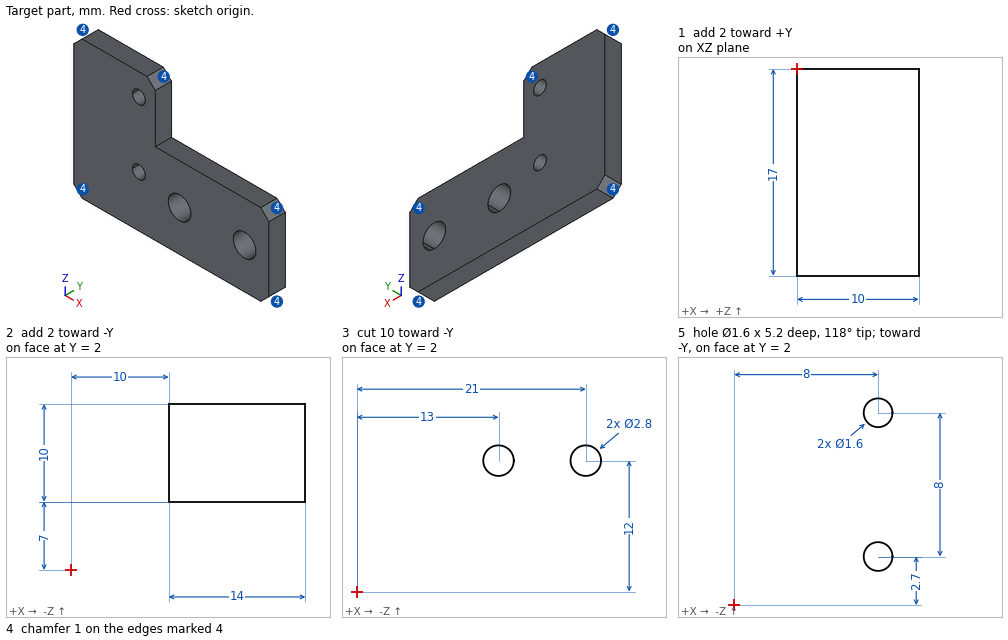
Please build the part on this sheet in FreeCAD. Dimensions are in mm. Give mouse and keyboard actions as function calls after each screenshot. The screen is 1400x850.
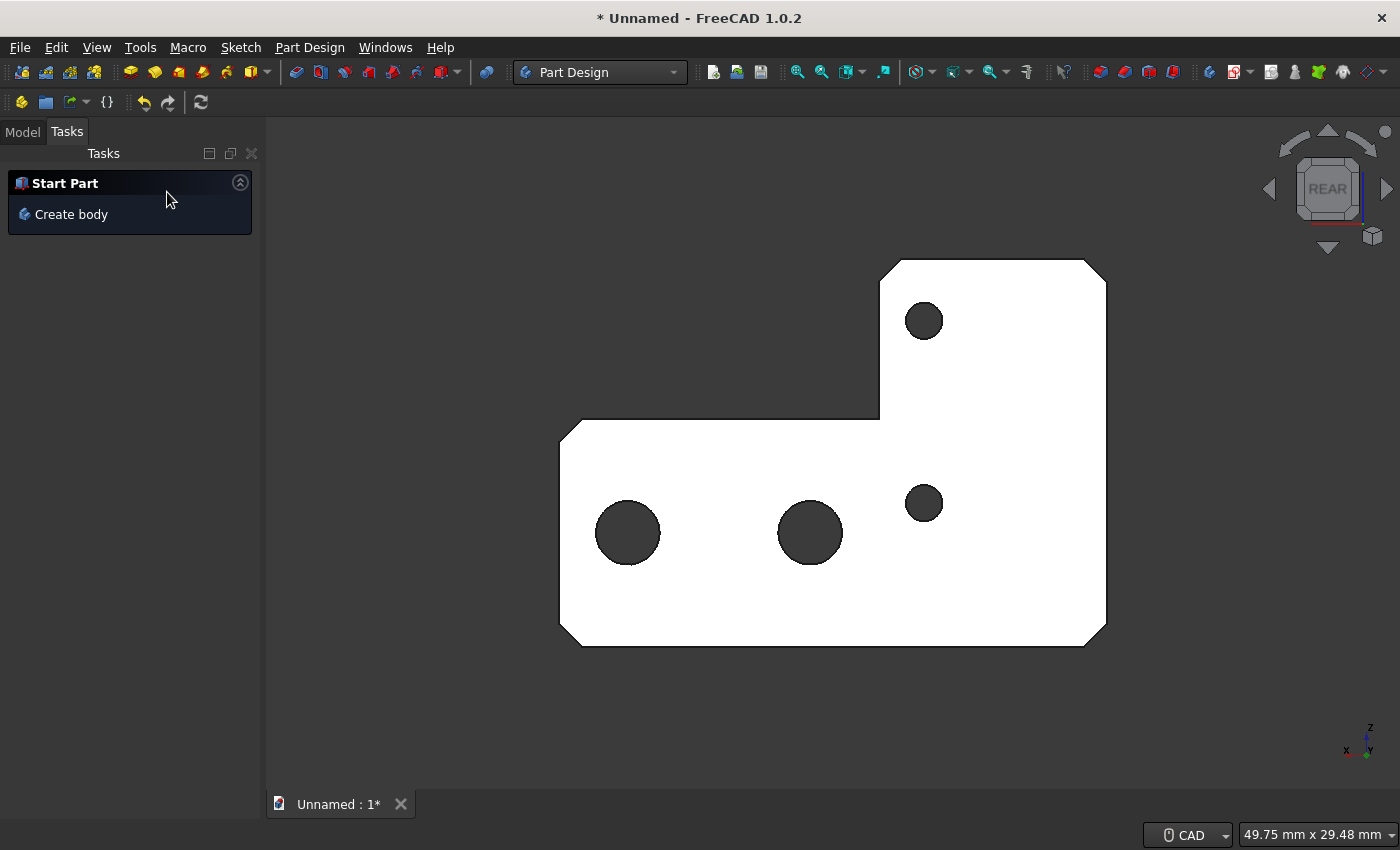
key(0)